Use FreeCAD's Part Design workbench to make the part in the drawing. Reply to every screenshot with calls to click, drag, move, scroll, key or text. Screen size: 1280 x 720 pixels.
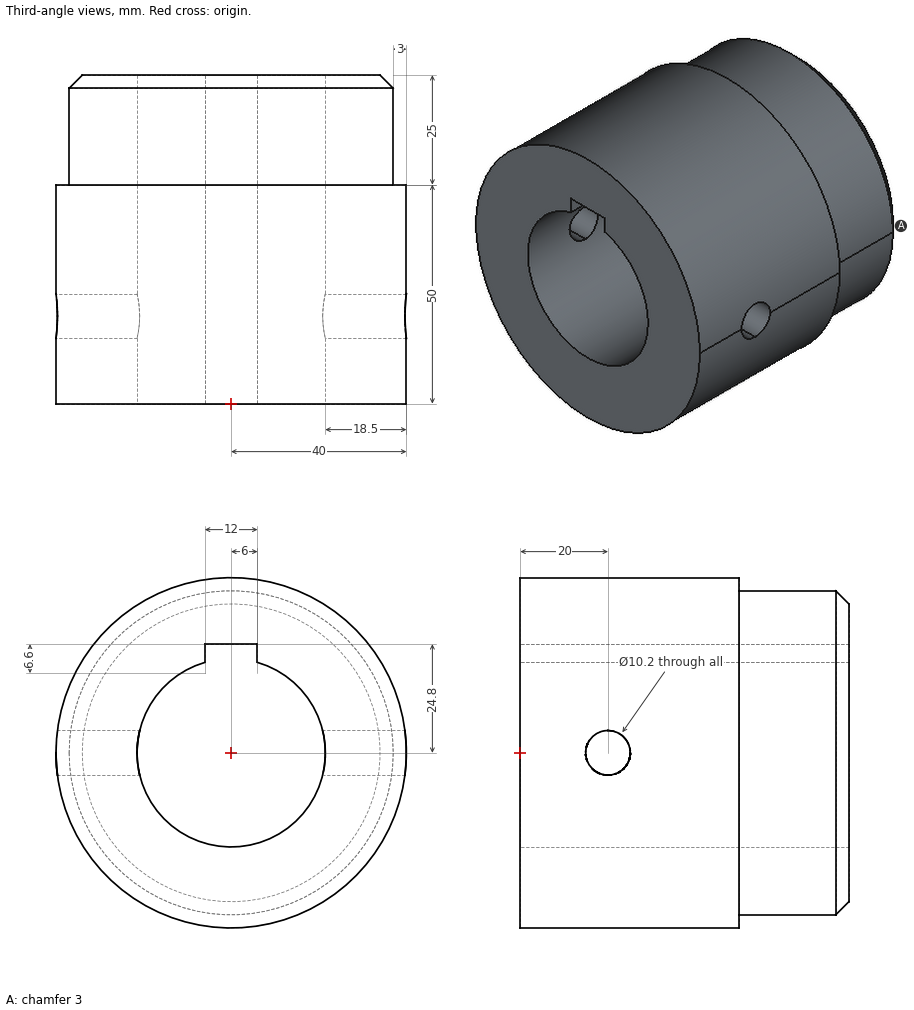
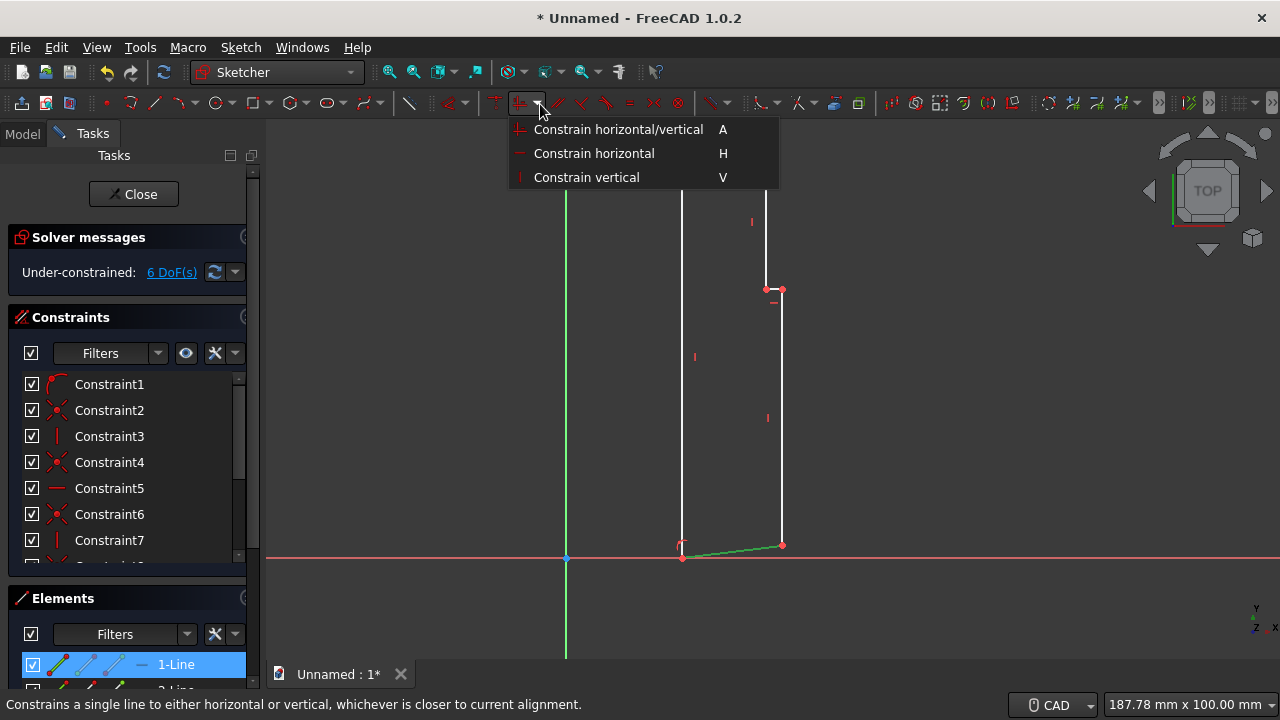
click(644, 153)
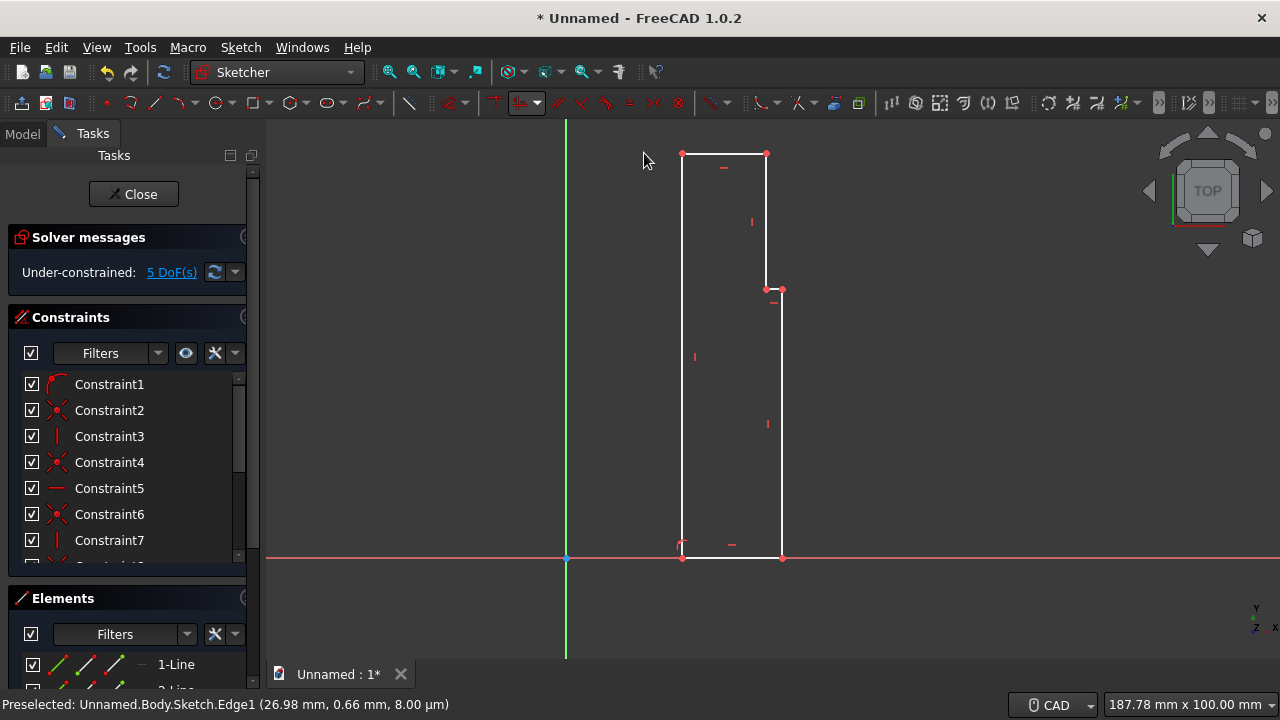
click(448, 104)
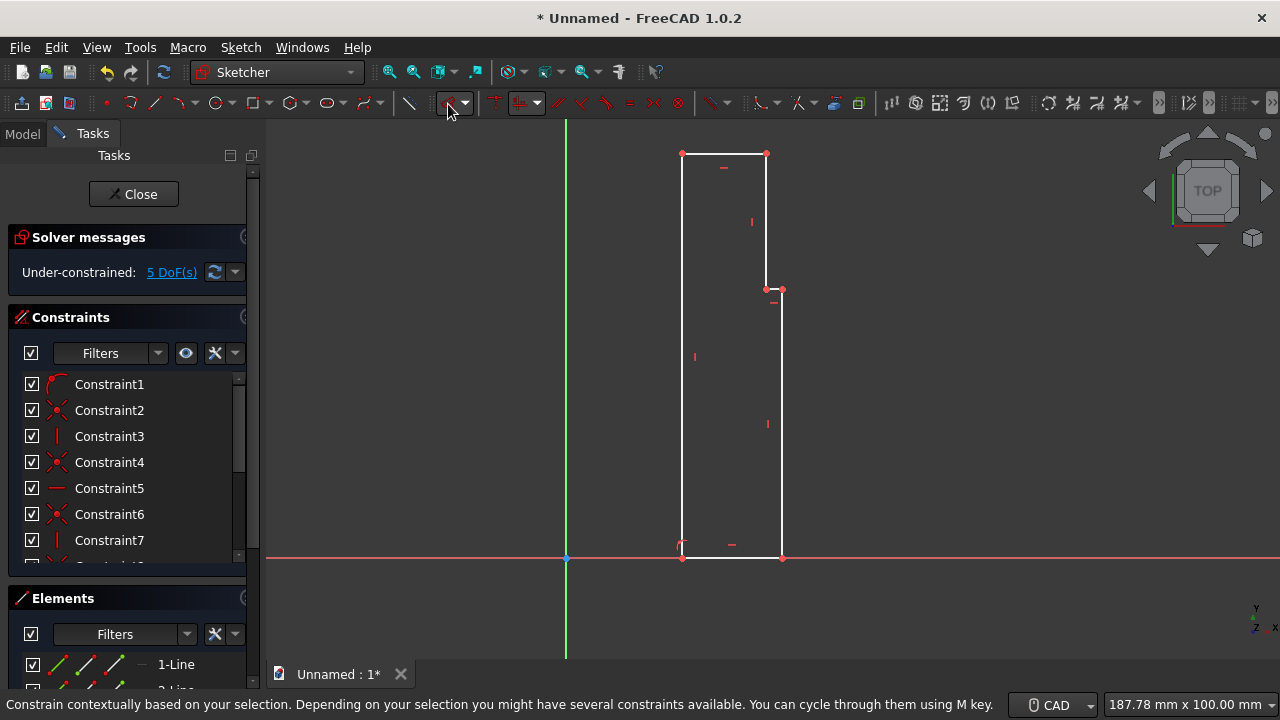
scroll(774, 289, up, 5)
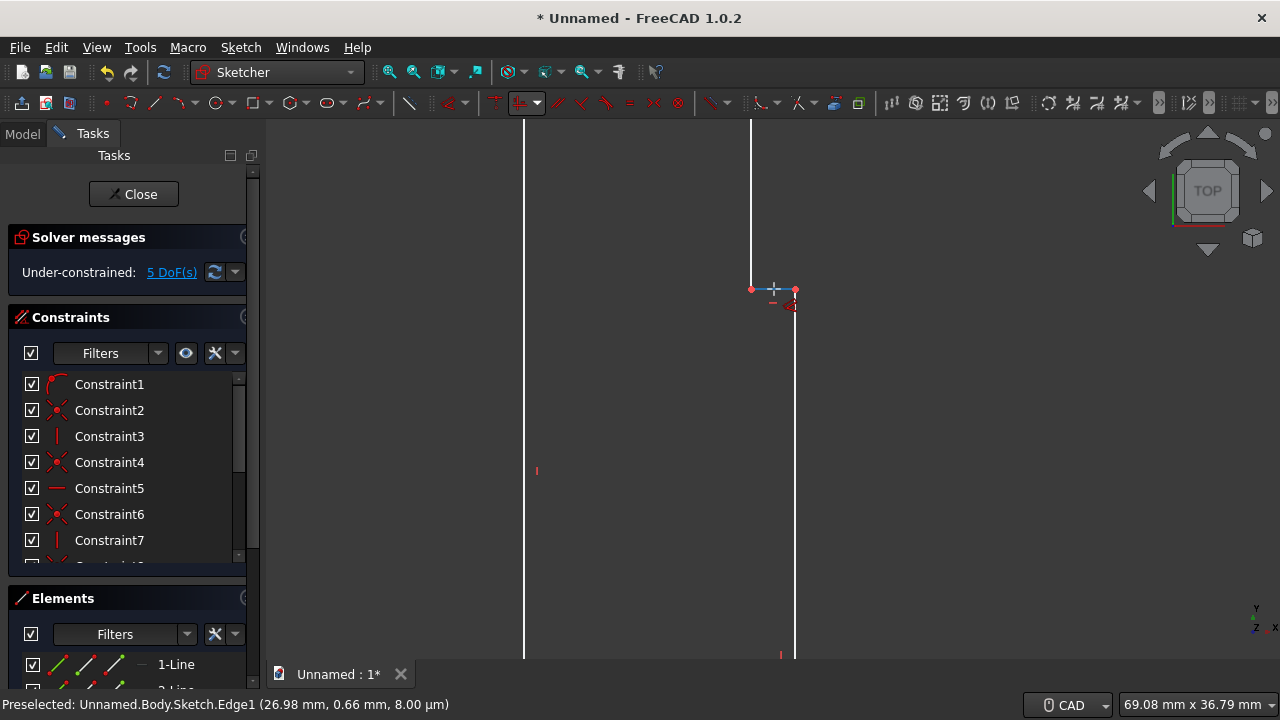
click(773, 289)
click(773, 255)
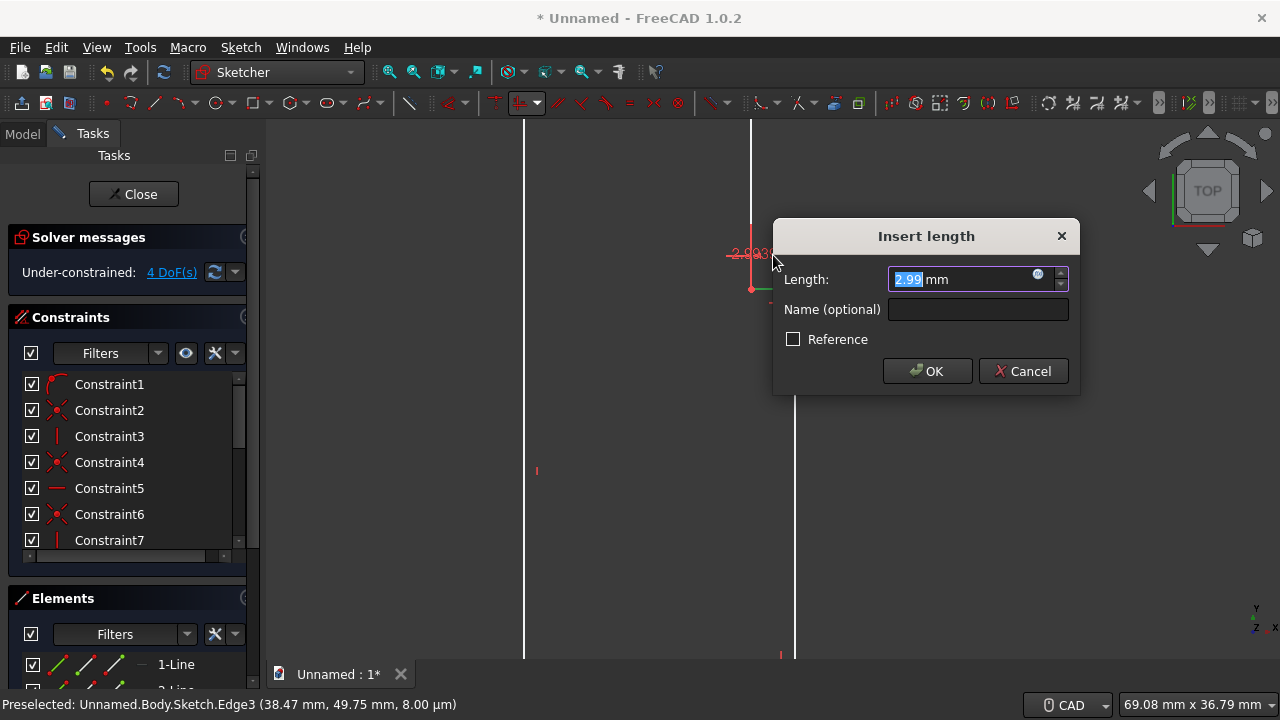
text(3)
key(Return)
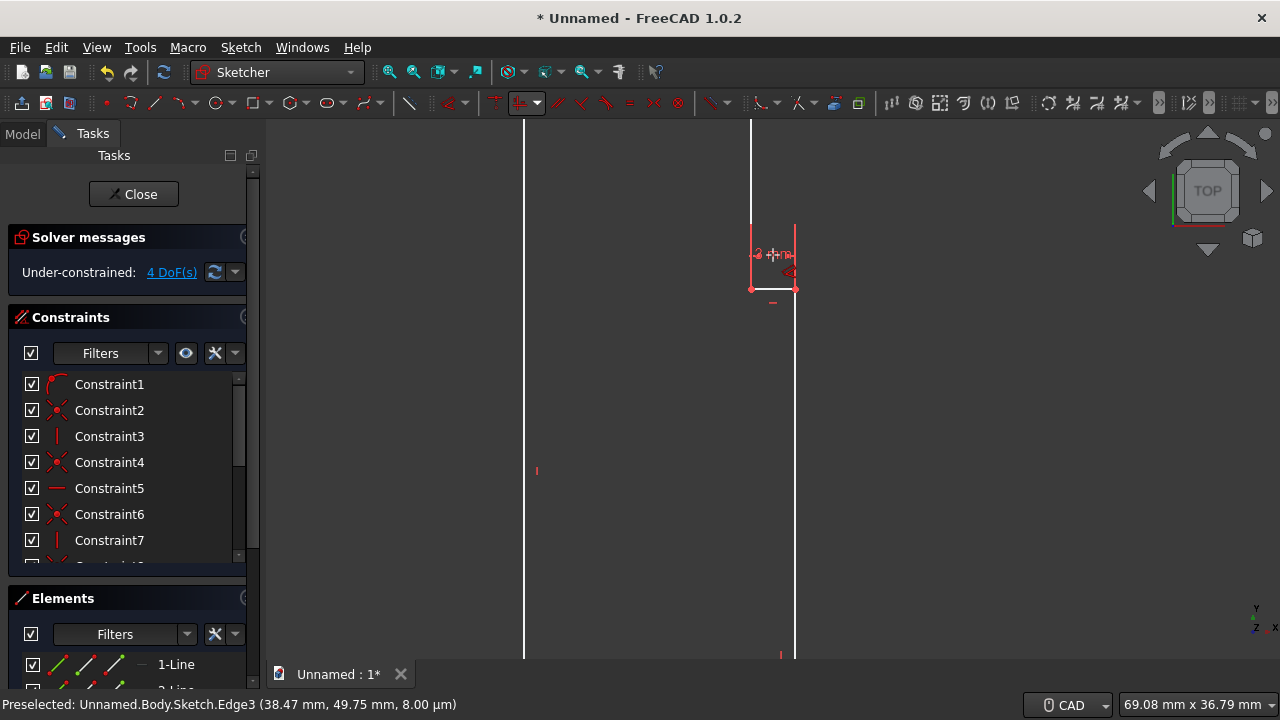
scroll(792, 354, down, 6)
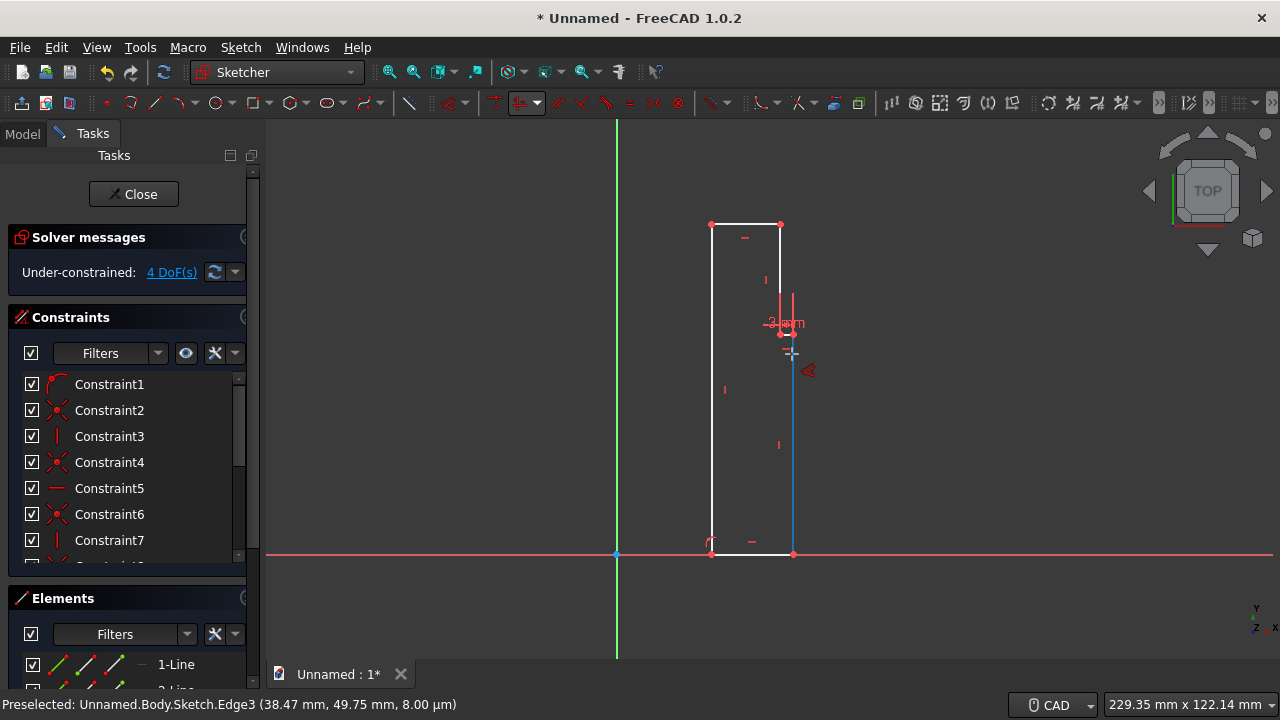
click(793, 401)
click(827, 445)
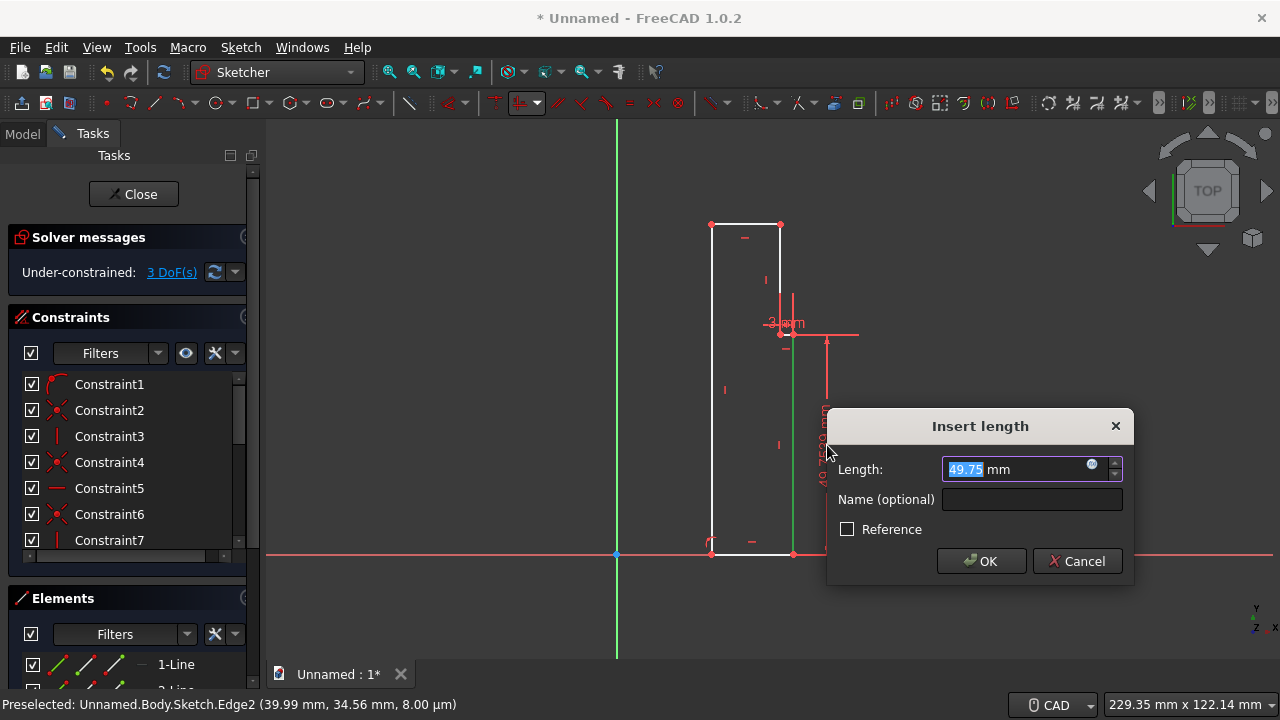
text(50)
key(Return)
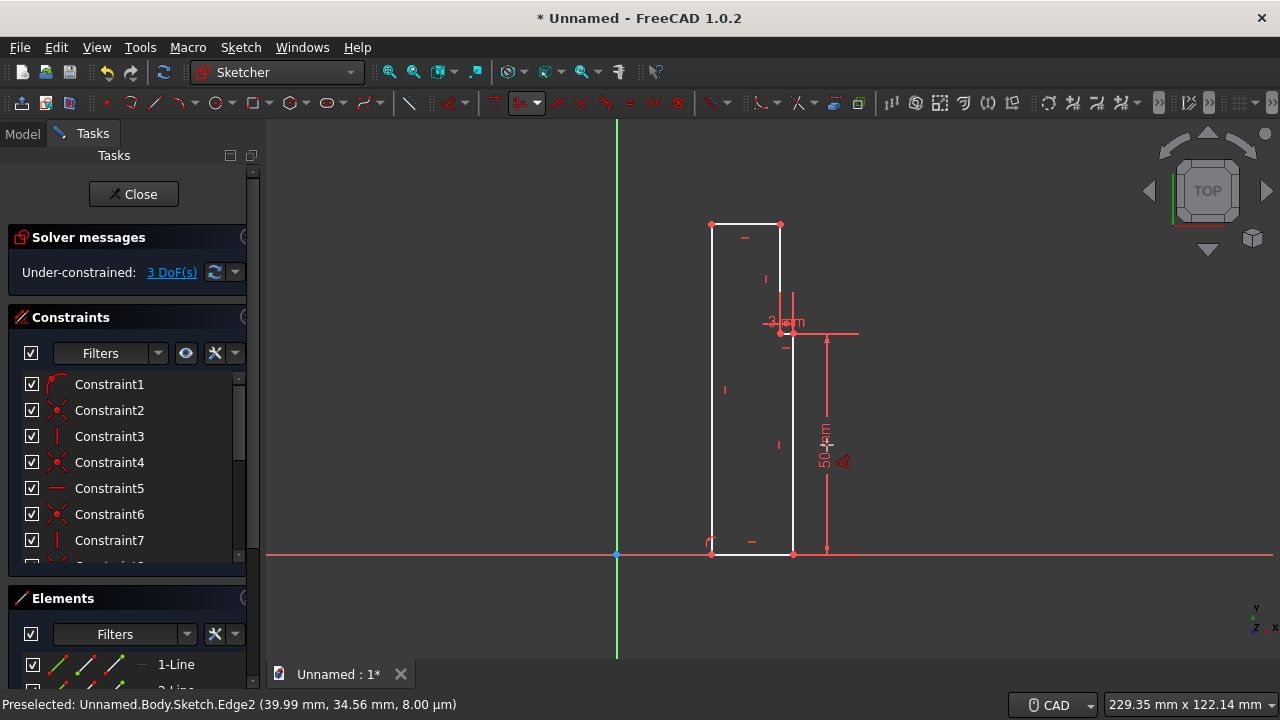
click(780, 301)
click(814, 279)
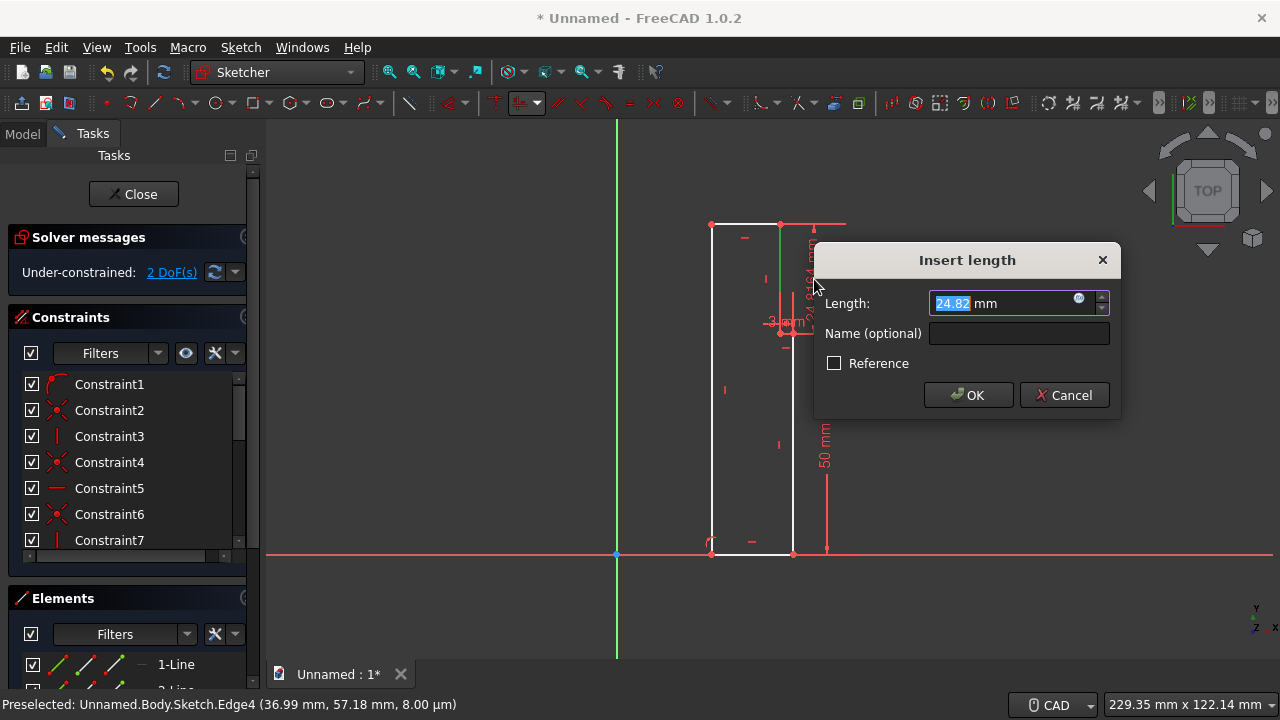
text(25)
key(Return)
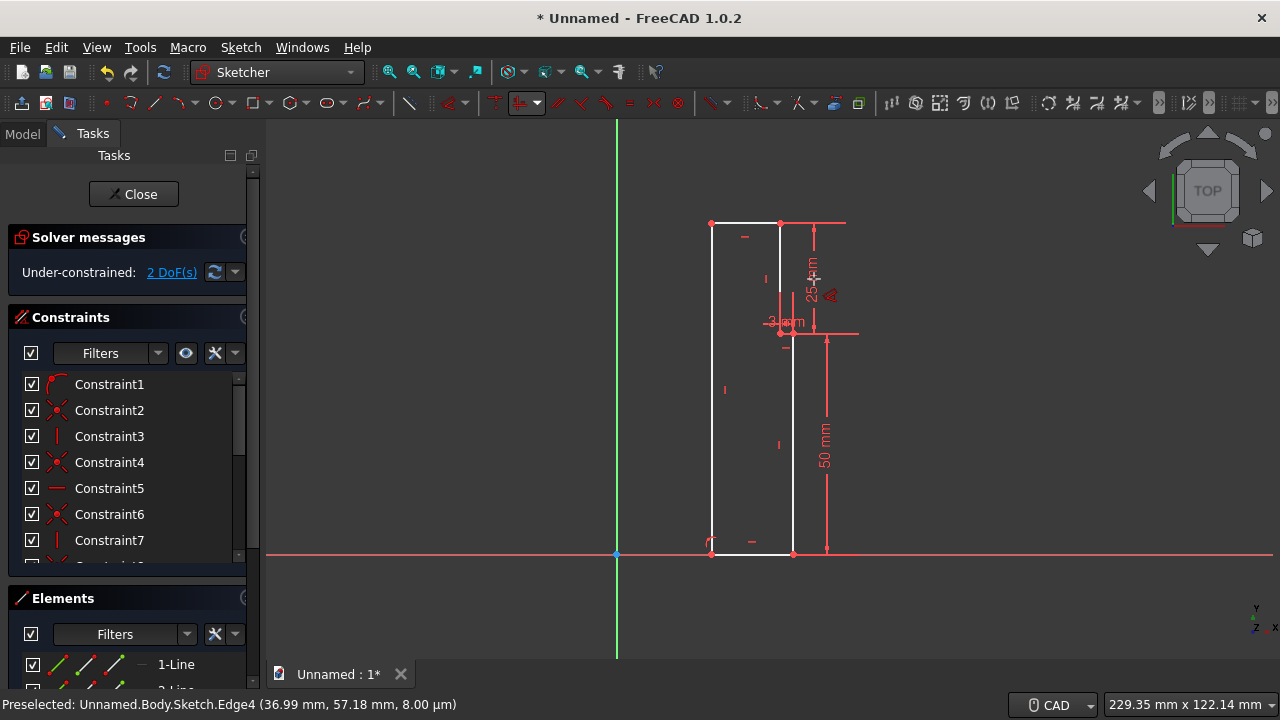
click(793, 555)
click(705, 589)